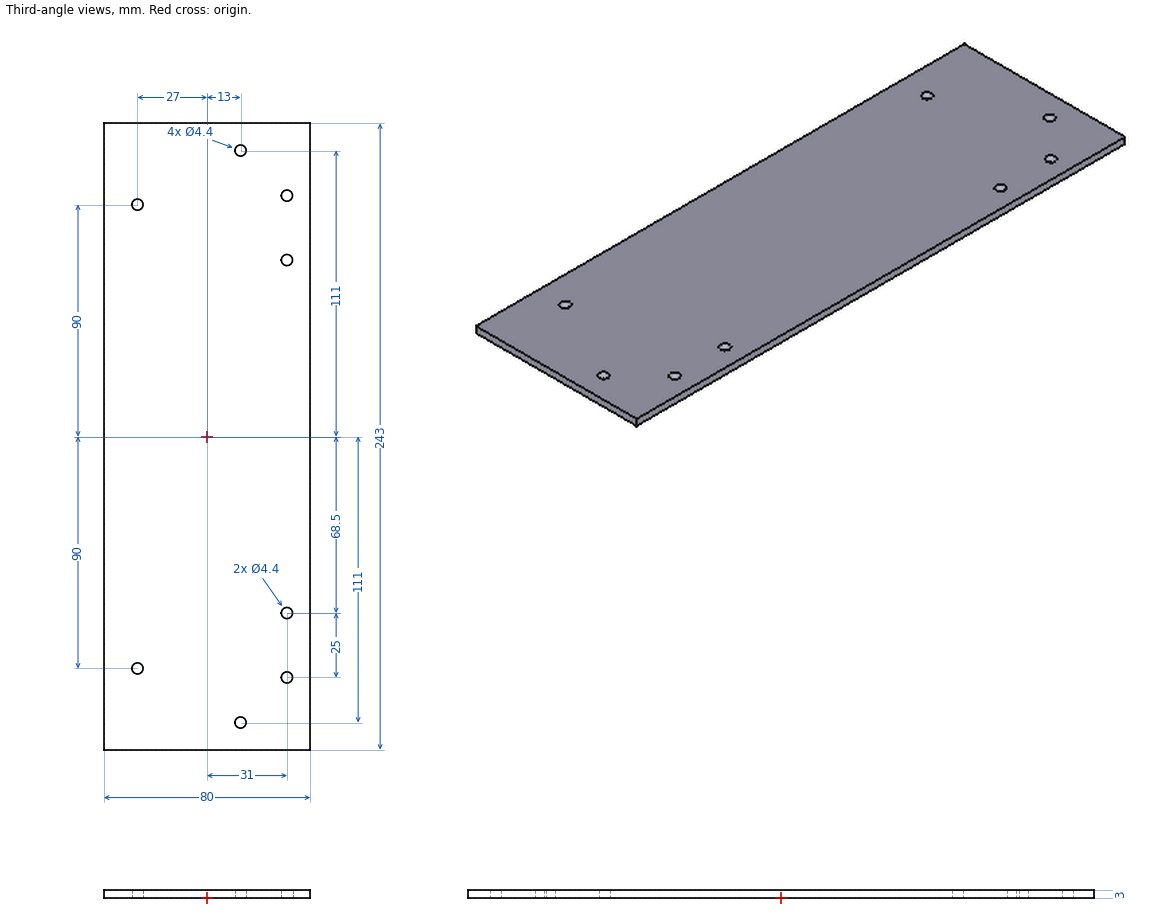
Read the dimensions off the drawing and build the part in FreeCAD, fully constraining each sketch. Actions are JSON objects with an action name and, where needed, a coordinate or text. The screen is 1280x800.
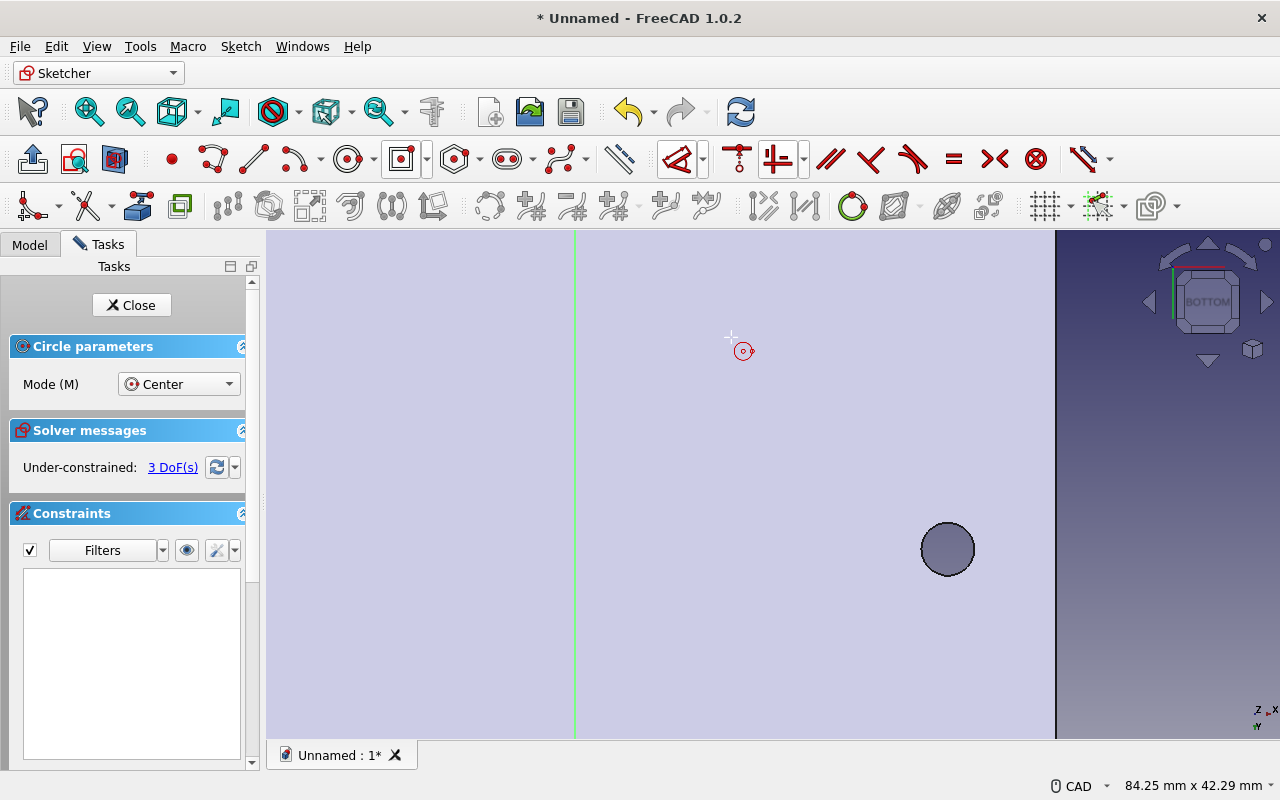
{"action": "scroll", "coordinate": [731, 336], "scroll_direction": "down", "scroll_amount": 11}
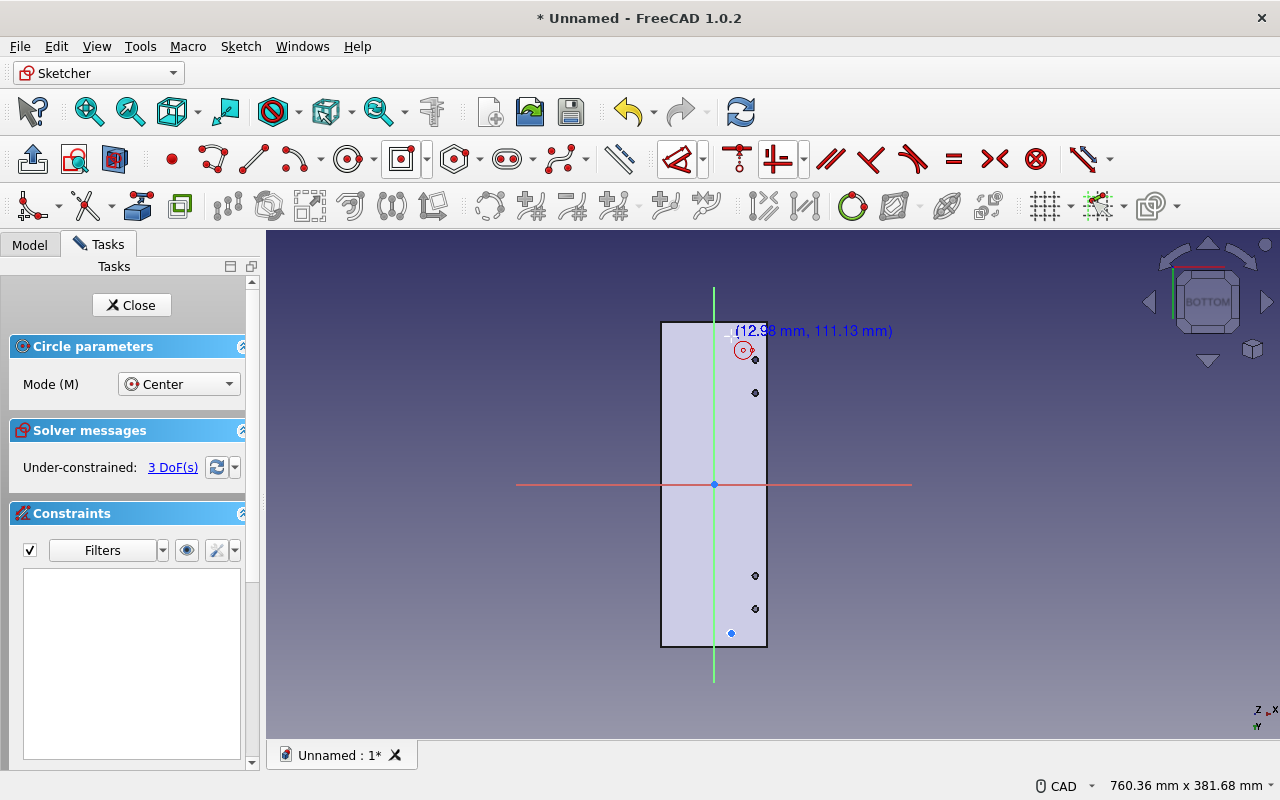
{"action": "left_click", "coordinate": [731, 336]}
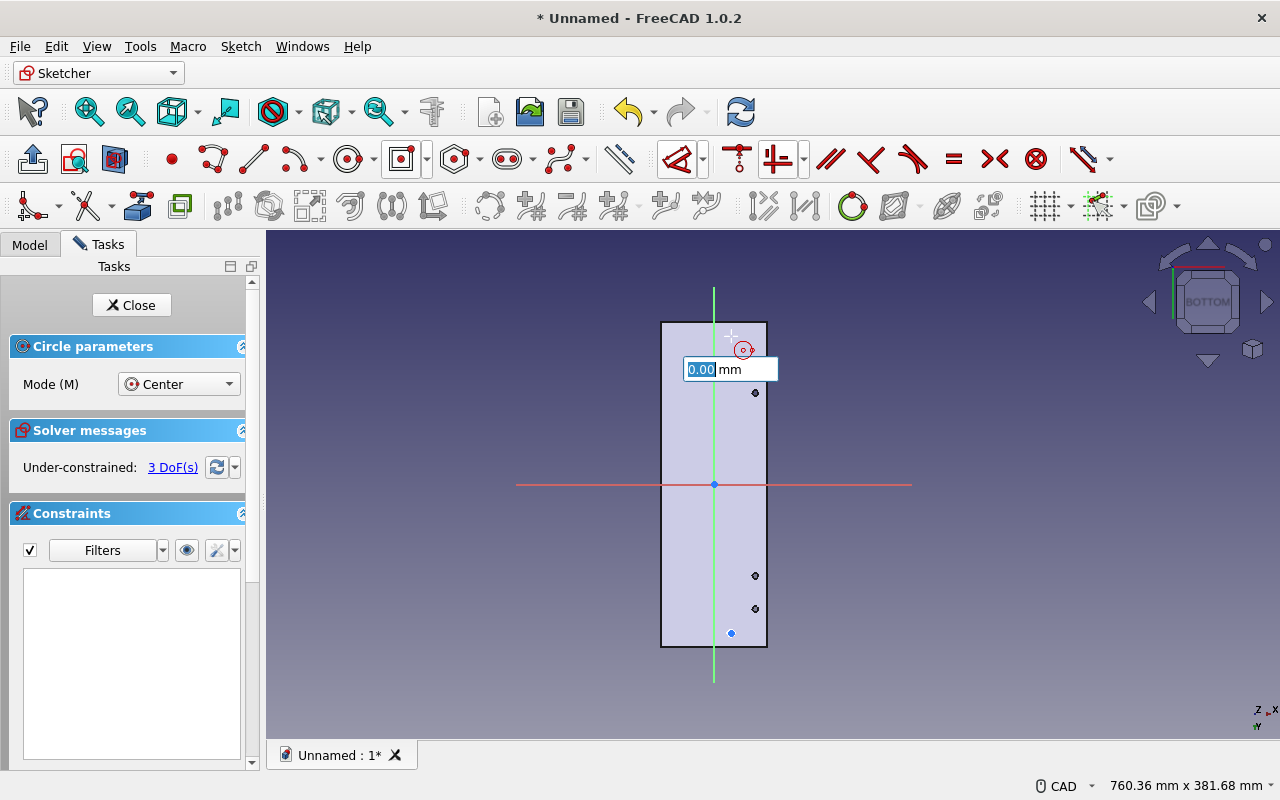
{"action": "scroll", "coordinate": [734, 334], "scroll_direction": "up", "scroll_amount": 9}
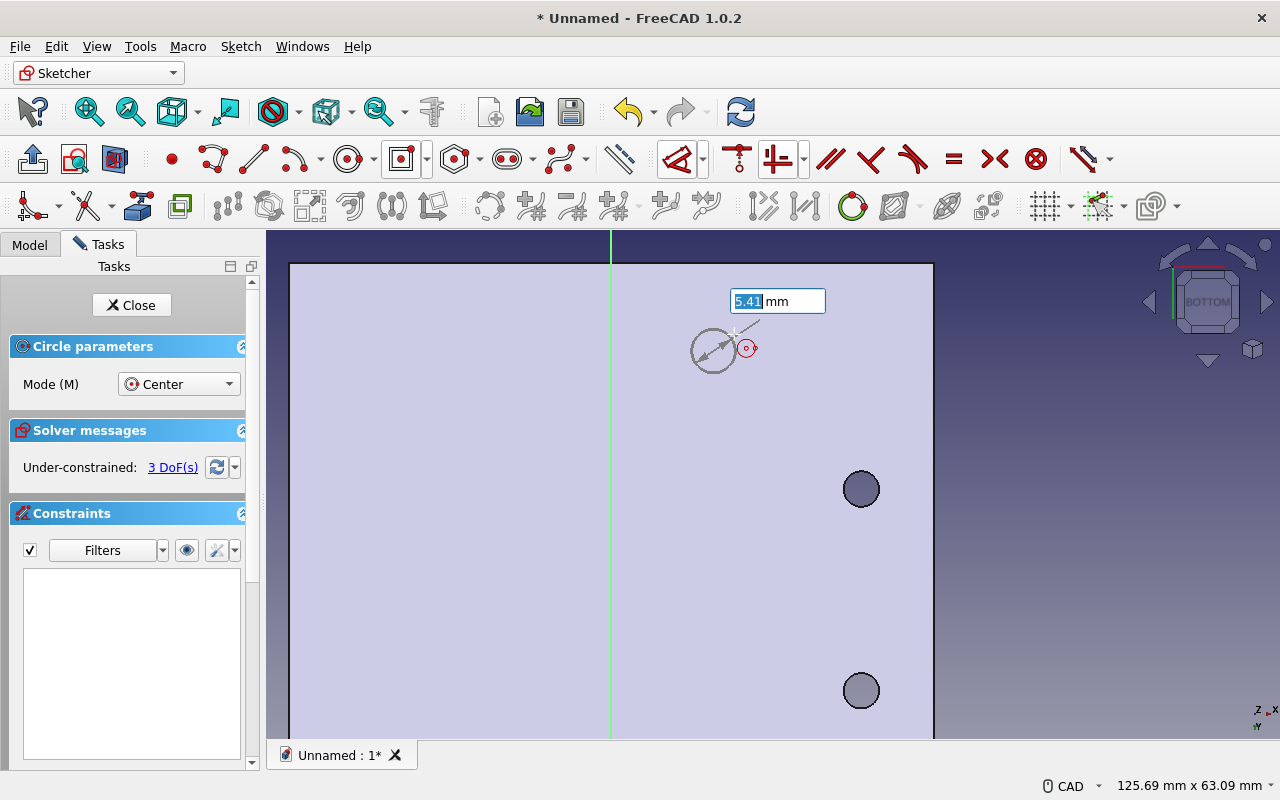
{"action": "left_click", "coordinate": [729, 335]}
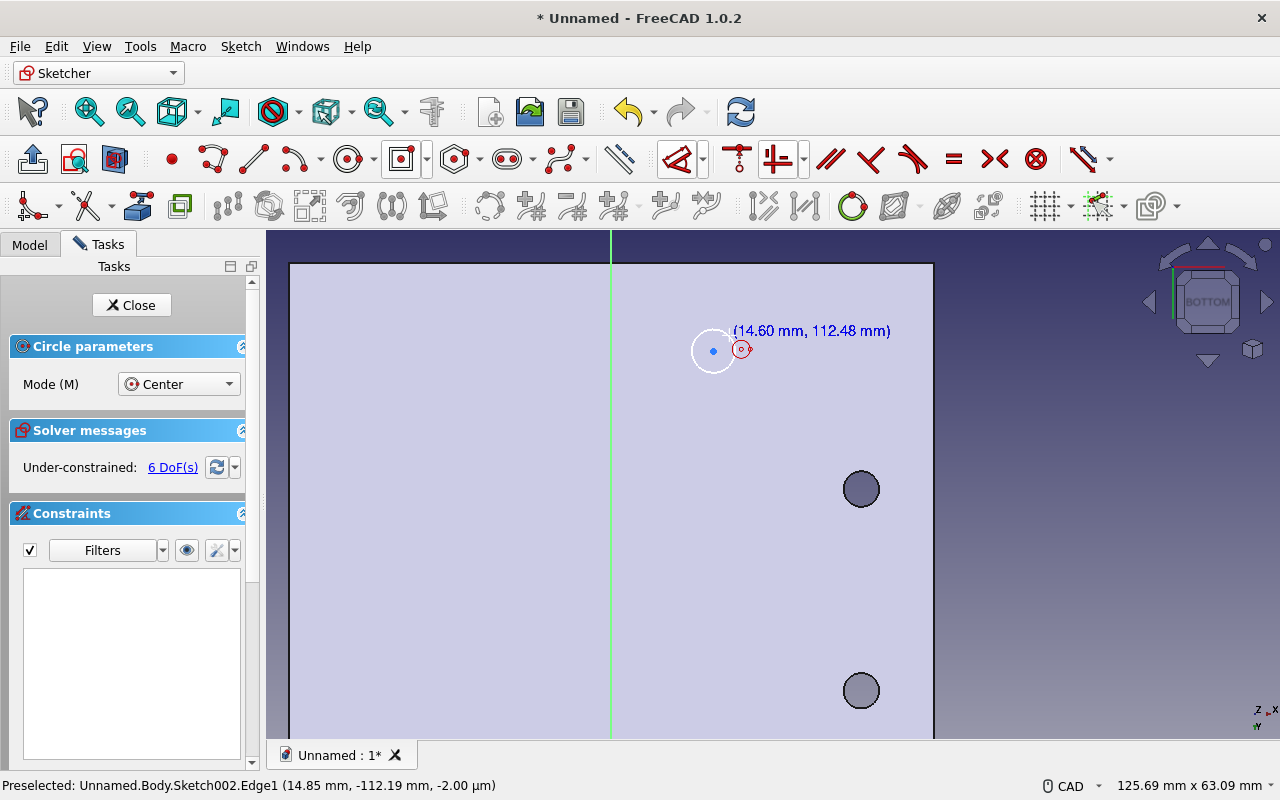
{"action": "scroll", "coordinate": [734, 334], "scroll_direction": "down", "scroll_amount": 9}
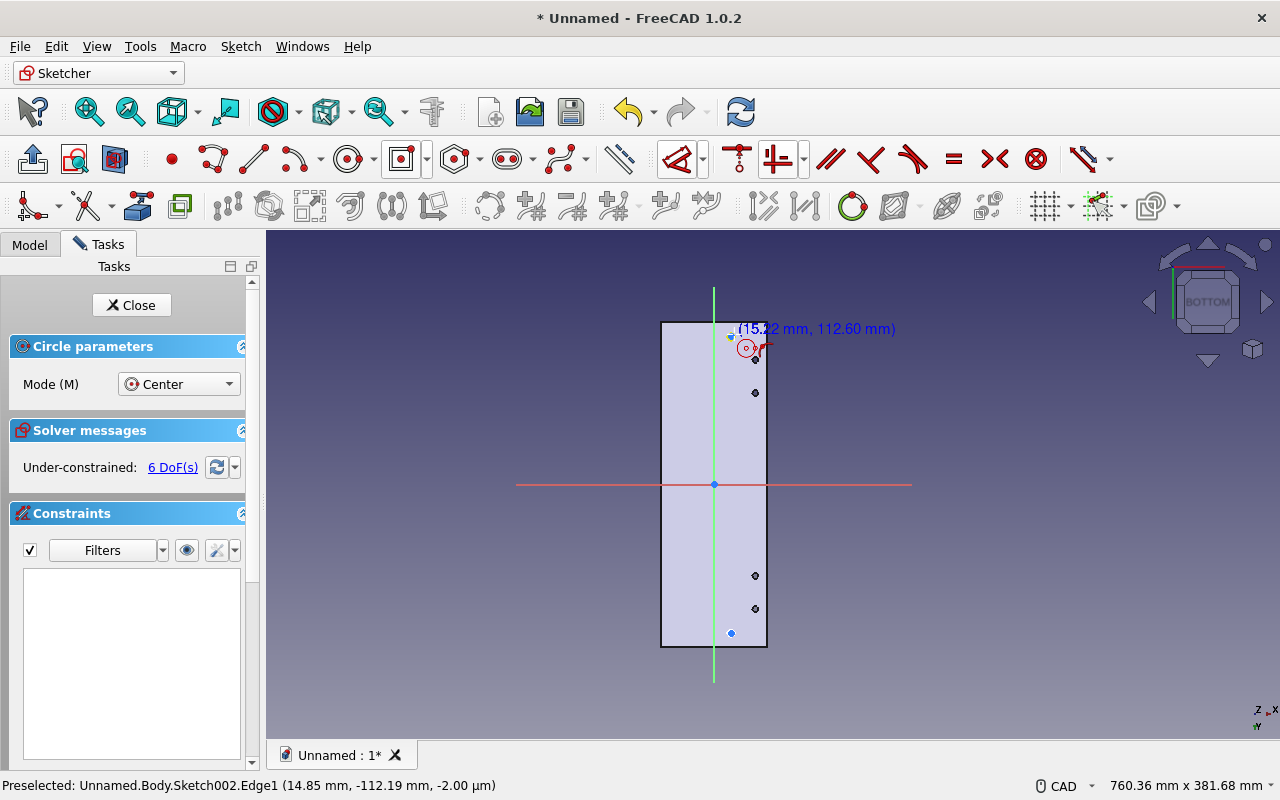
{"action": "scroll", "coordinate": [678, 605], "scroll_direction": "up", "scroll_amount": 11}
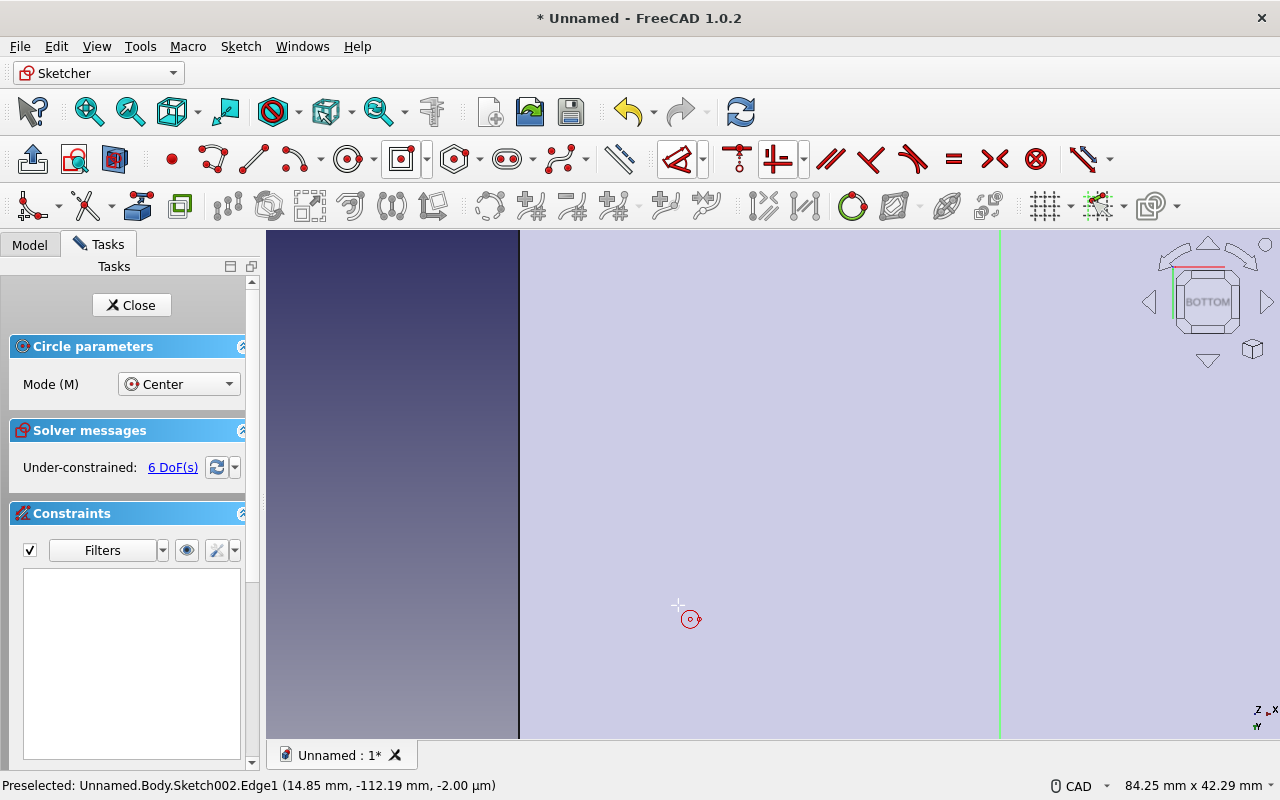
{"action": "scroll", "coordinate": [678, 606], "scroll_direction": "down", "scroll_amount": 11}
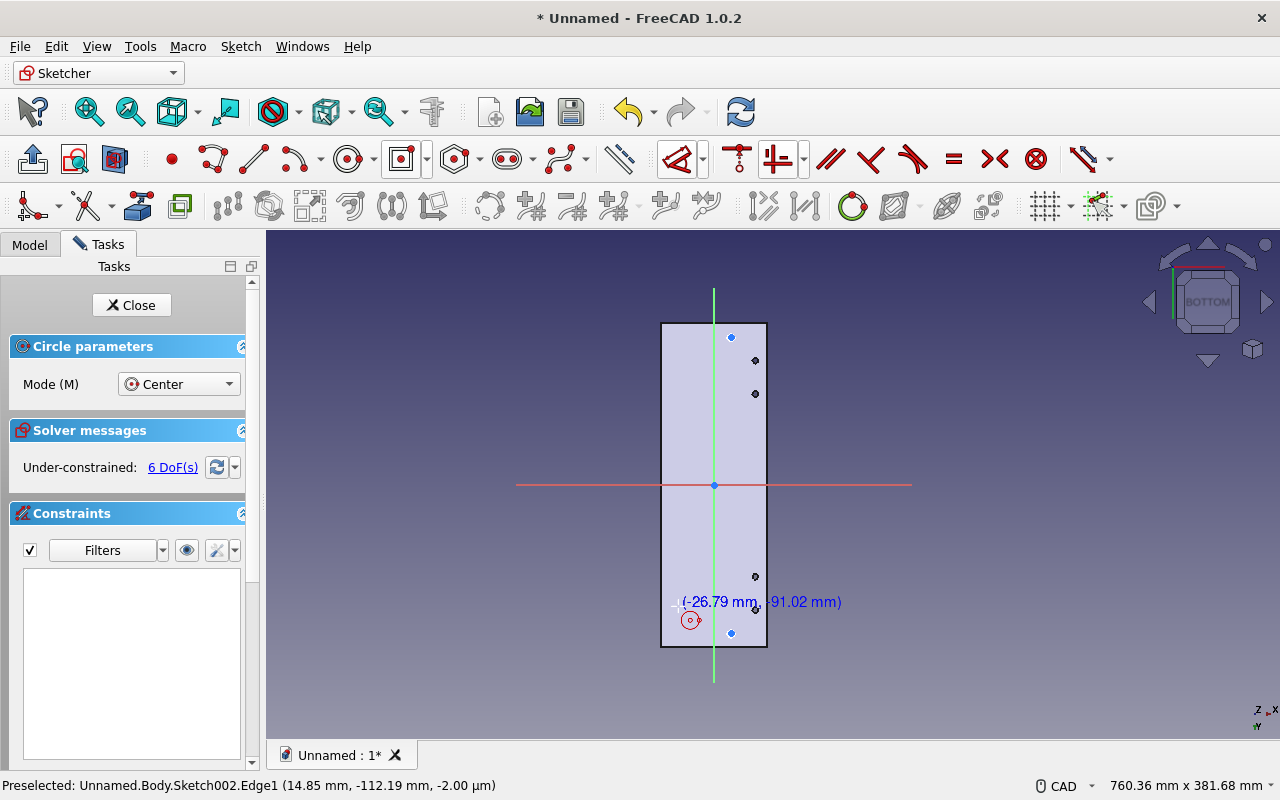
{"action": "left_click", "coordinate": [678, 605]}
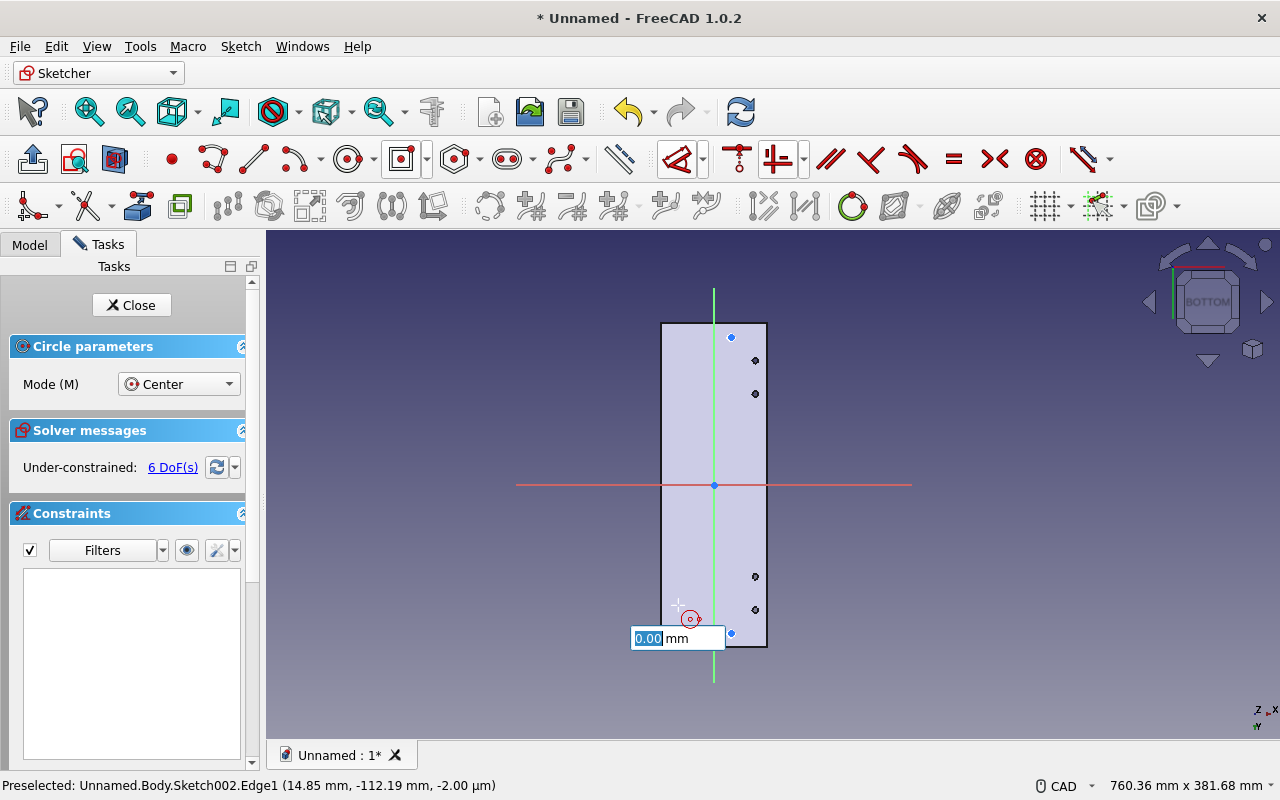
{"action": "scroll", "coordinate": [680, 603], "scroll_direction": "up", "scroll_amount": 9}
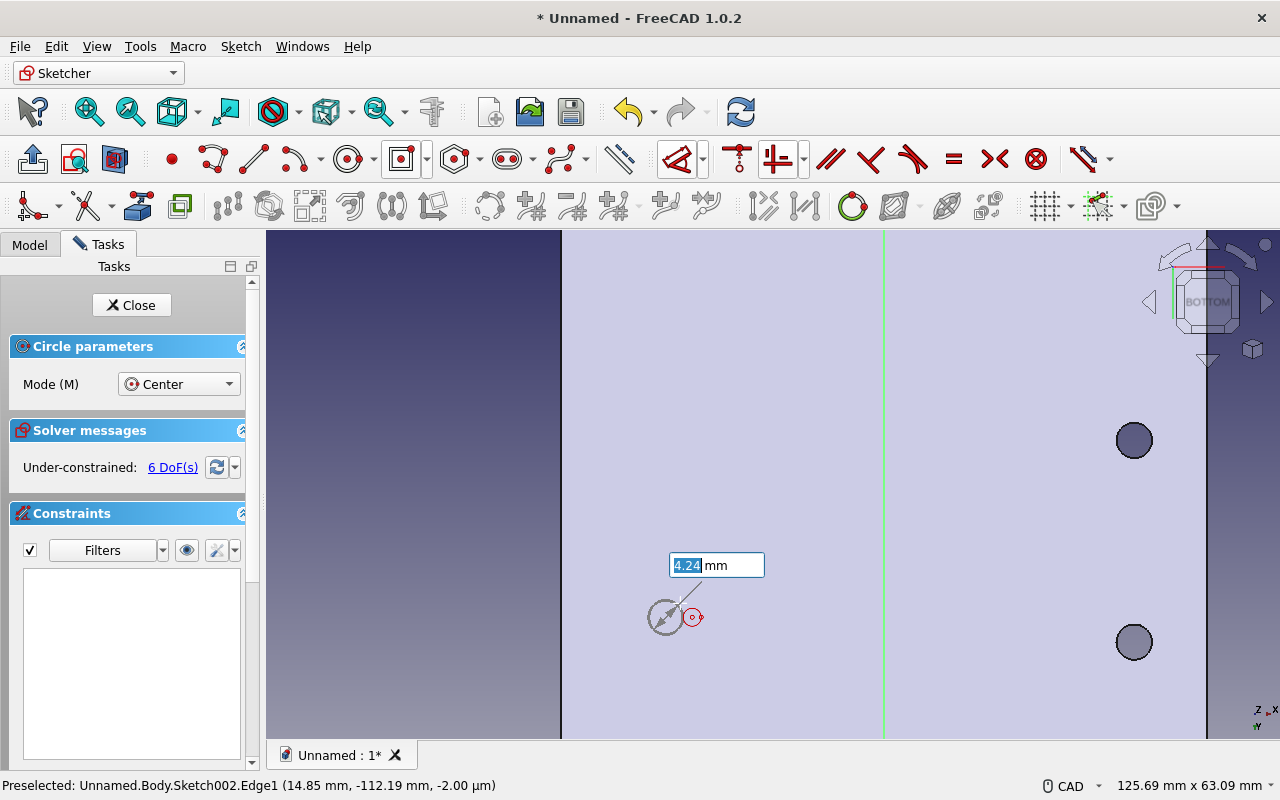
{"action": "left_click", "coordinate": [679, 601]}